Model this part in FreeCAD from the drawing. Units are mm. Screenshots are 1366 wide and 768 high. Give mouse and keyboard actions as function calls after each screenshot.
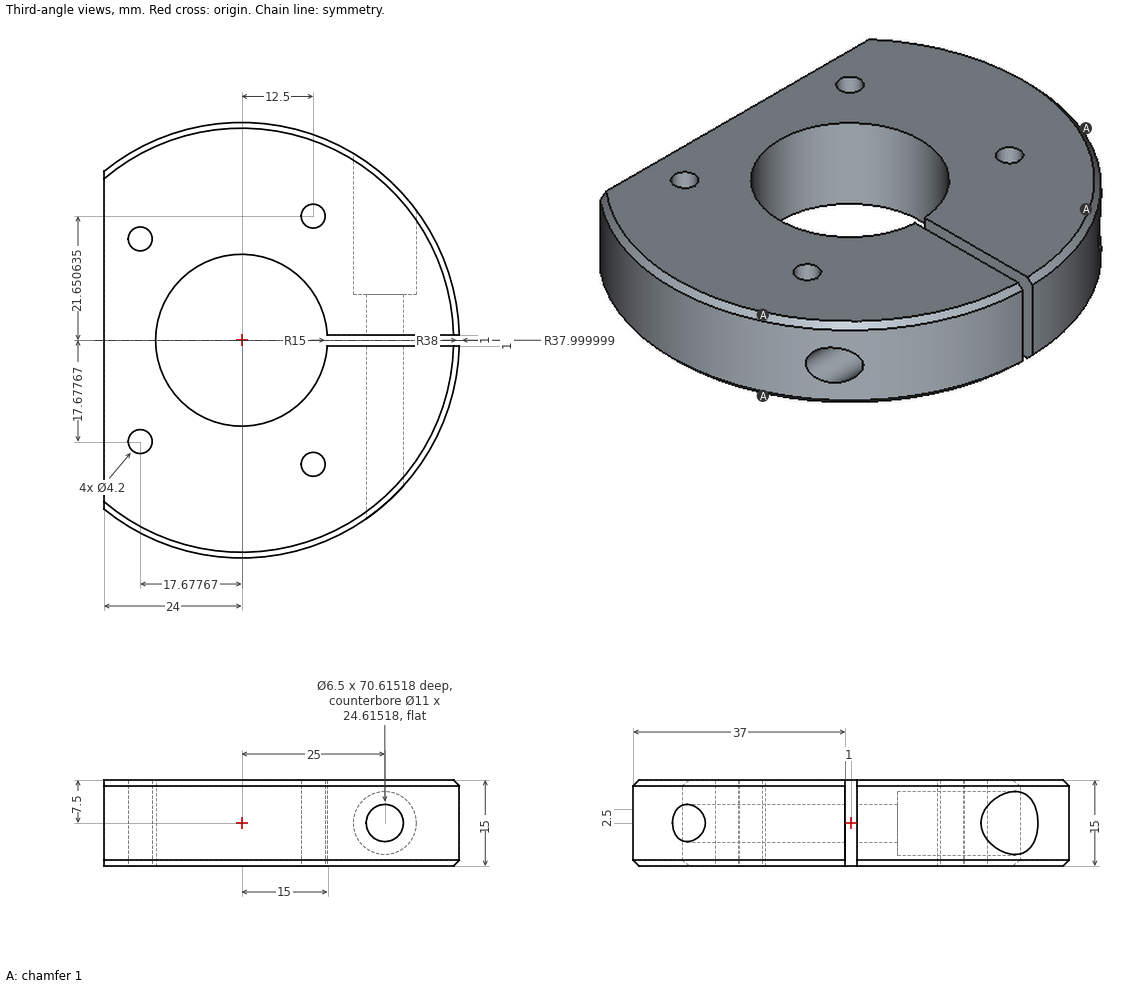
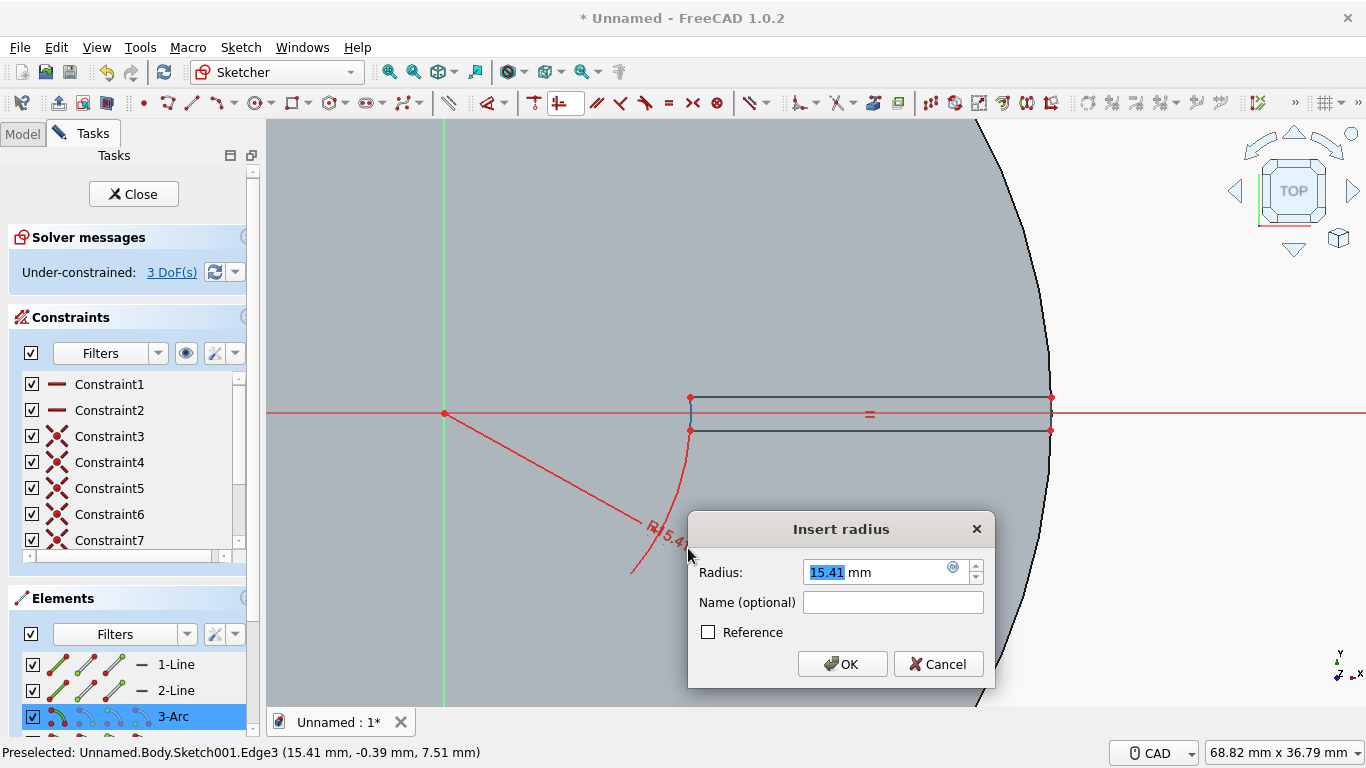
text(15)
key(Return)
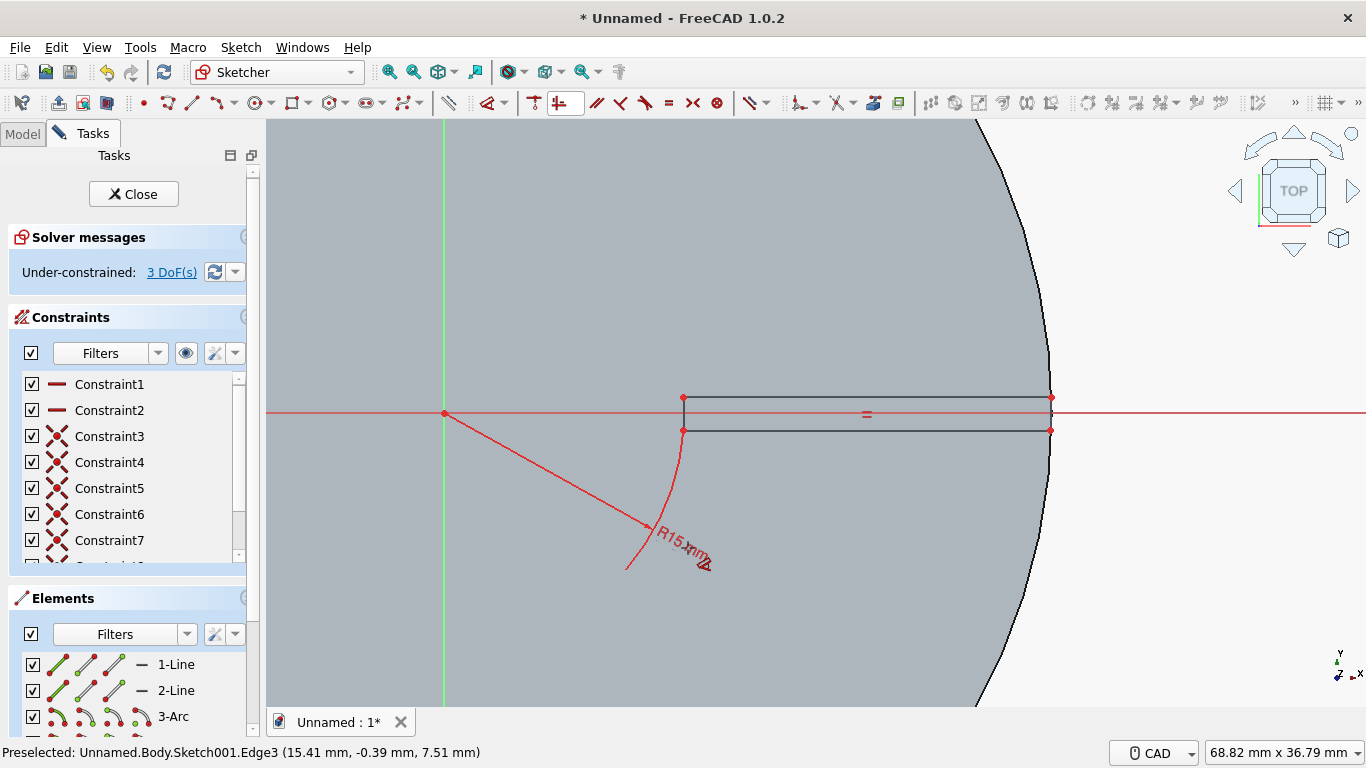
click(1051, 414)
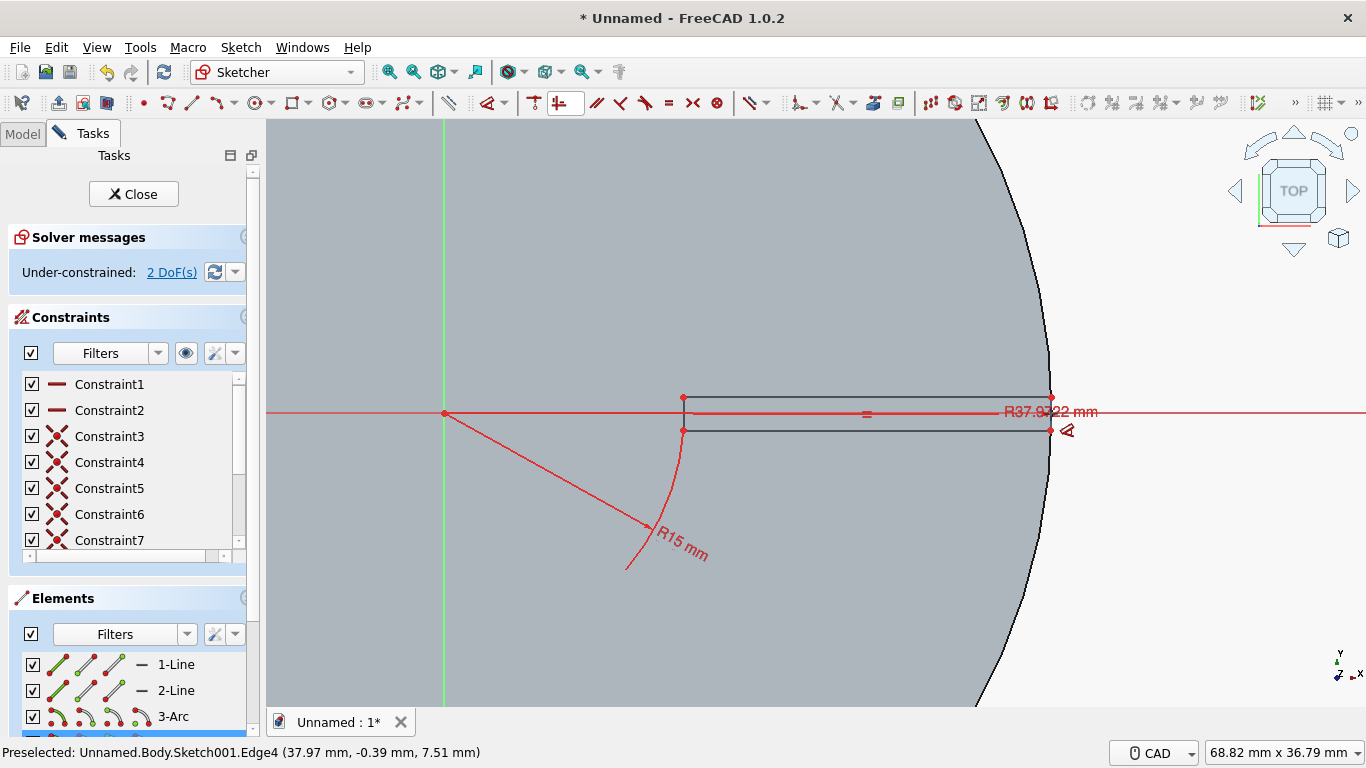
key(Escape)
key(Escape)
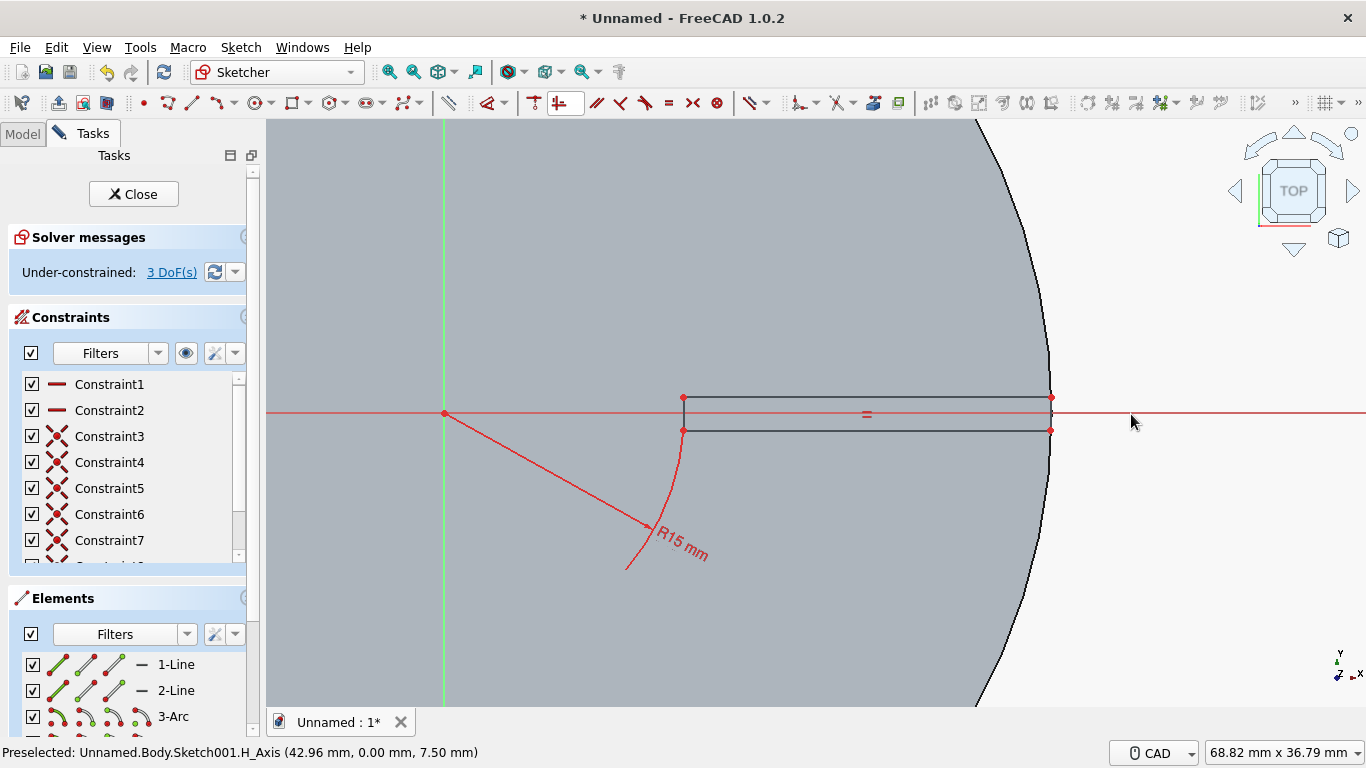
click(1051, 414)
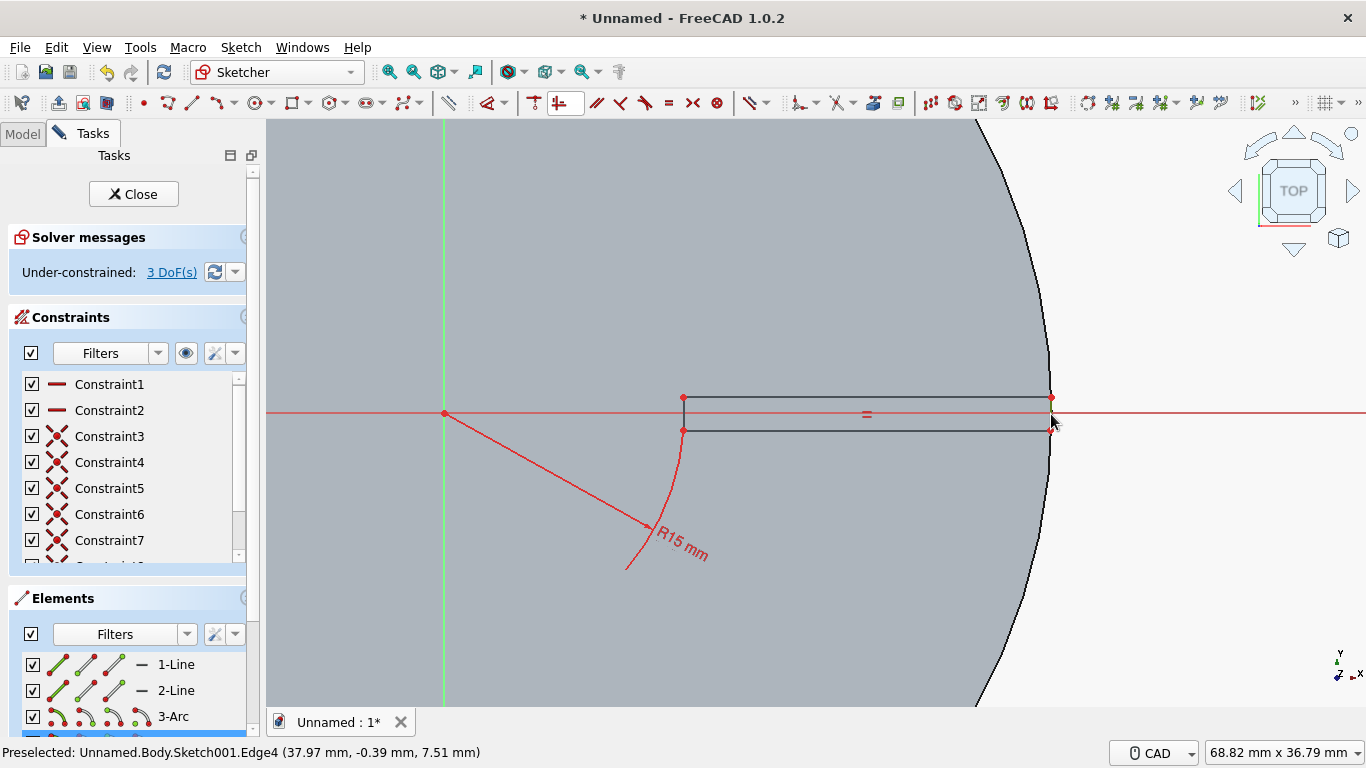
click(506, 104)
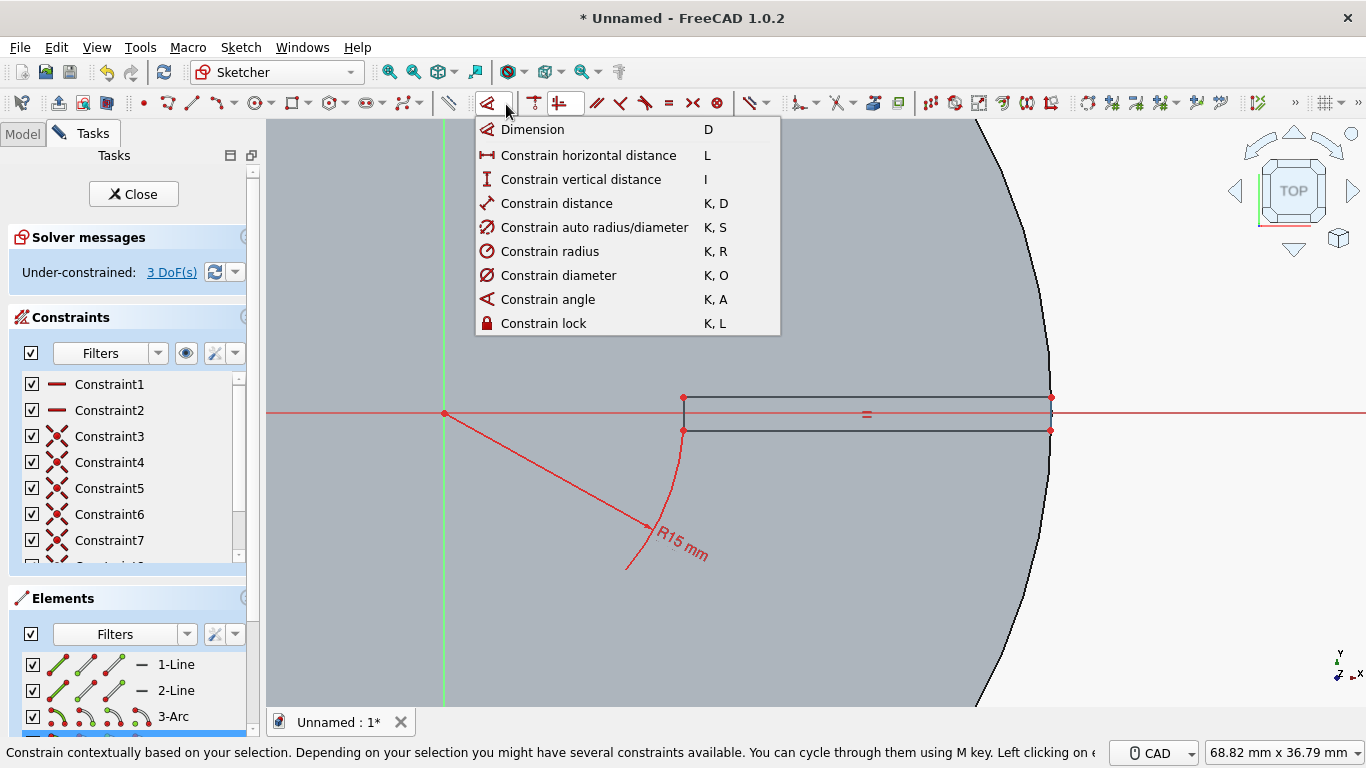
click(628, 251)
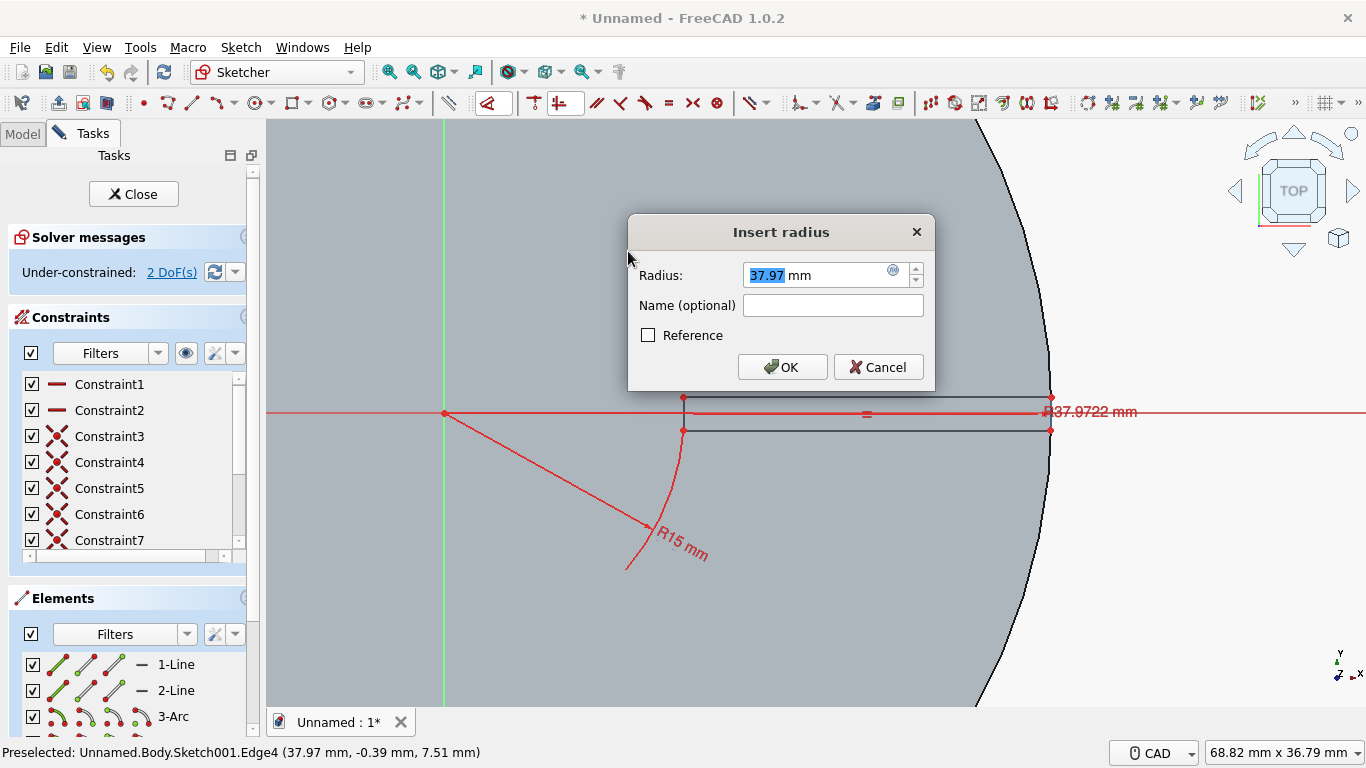
text(37.999999)
key(Return)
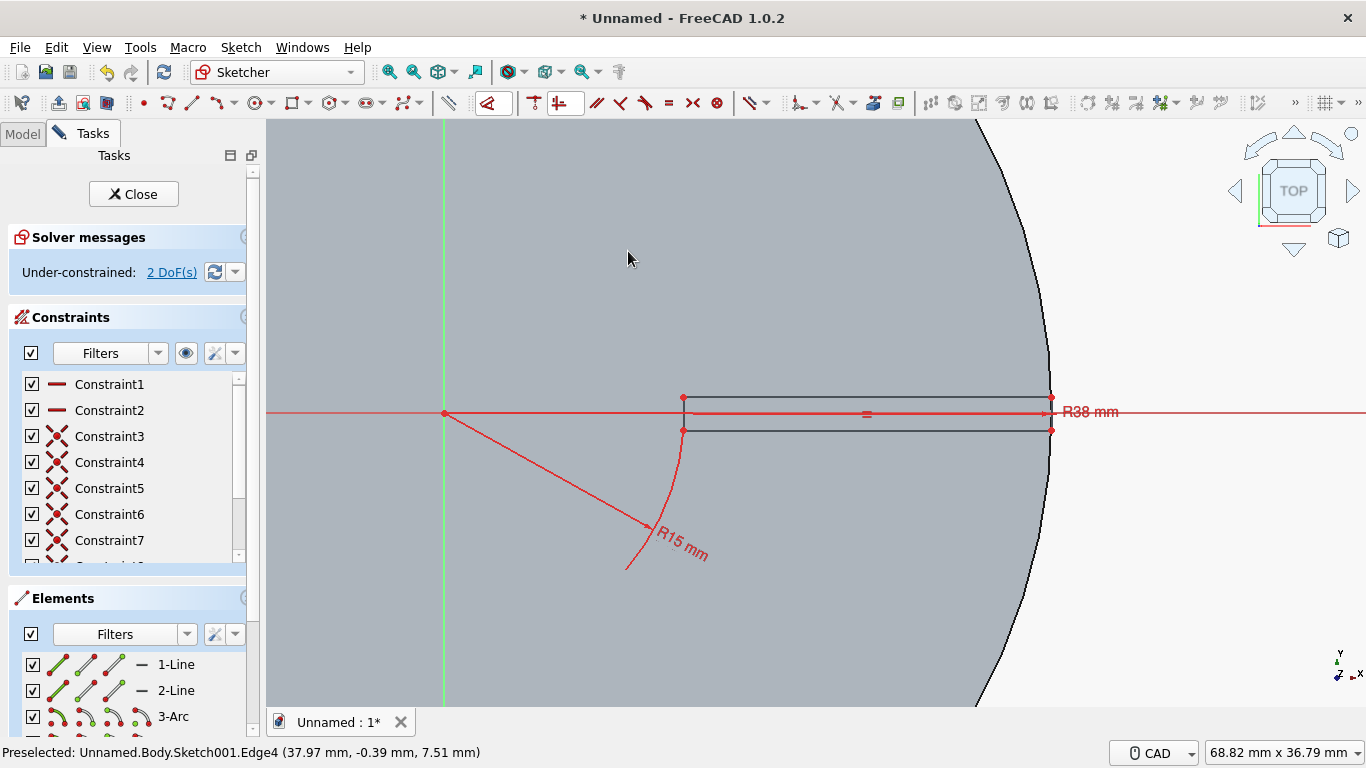
scroll(1051, 397, up, 14)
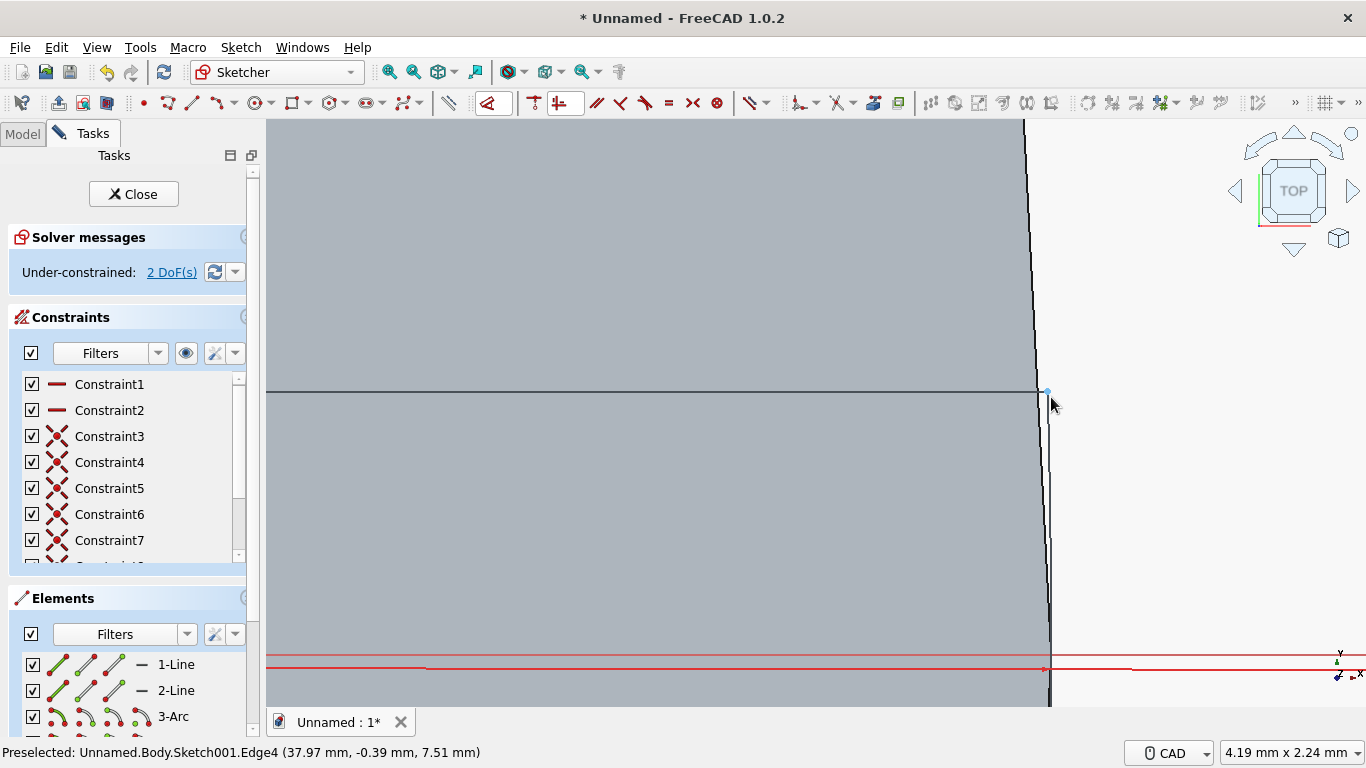
click(1048, 392)